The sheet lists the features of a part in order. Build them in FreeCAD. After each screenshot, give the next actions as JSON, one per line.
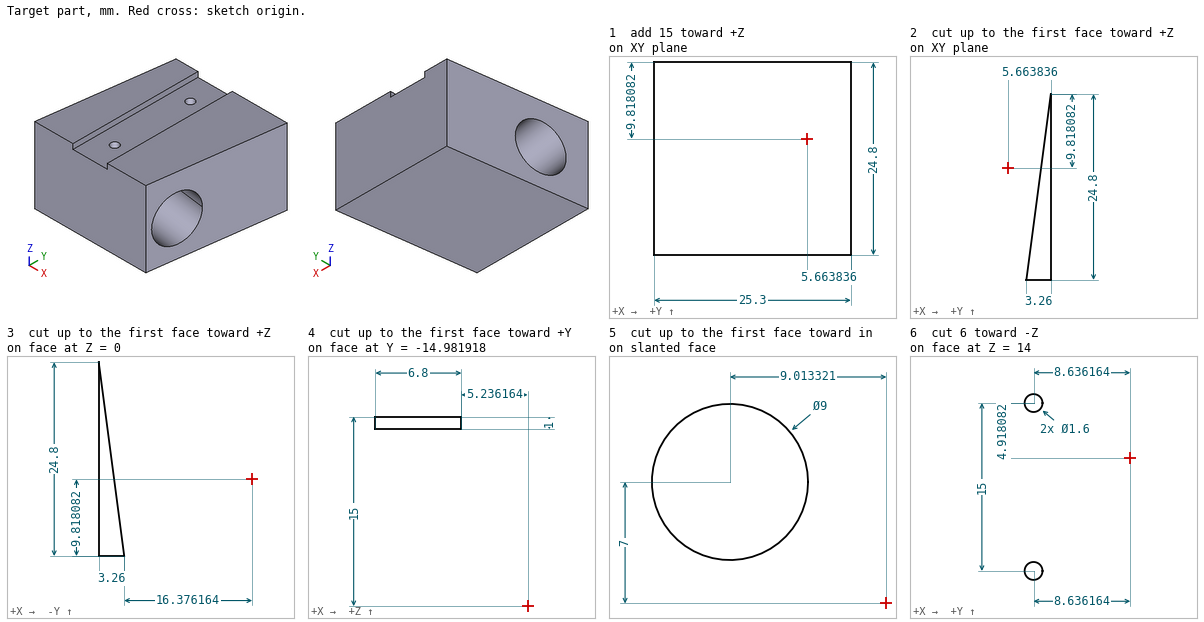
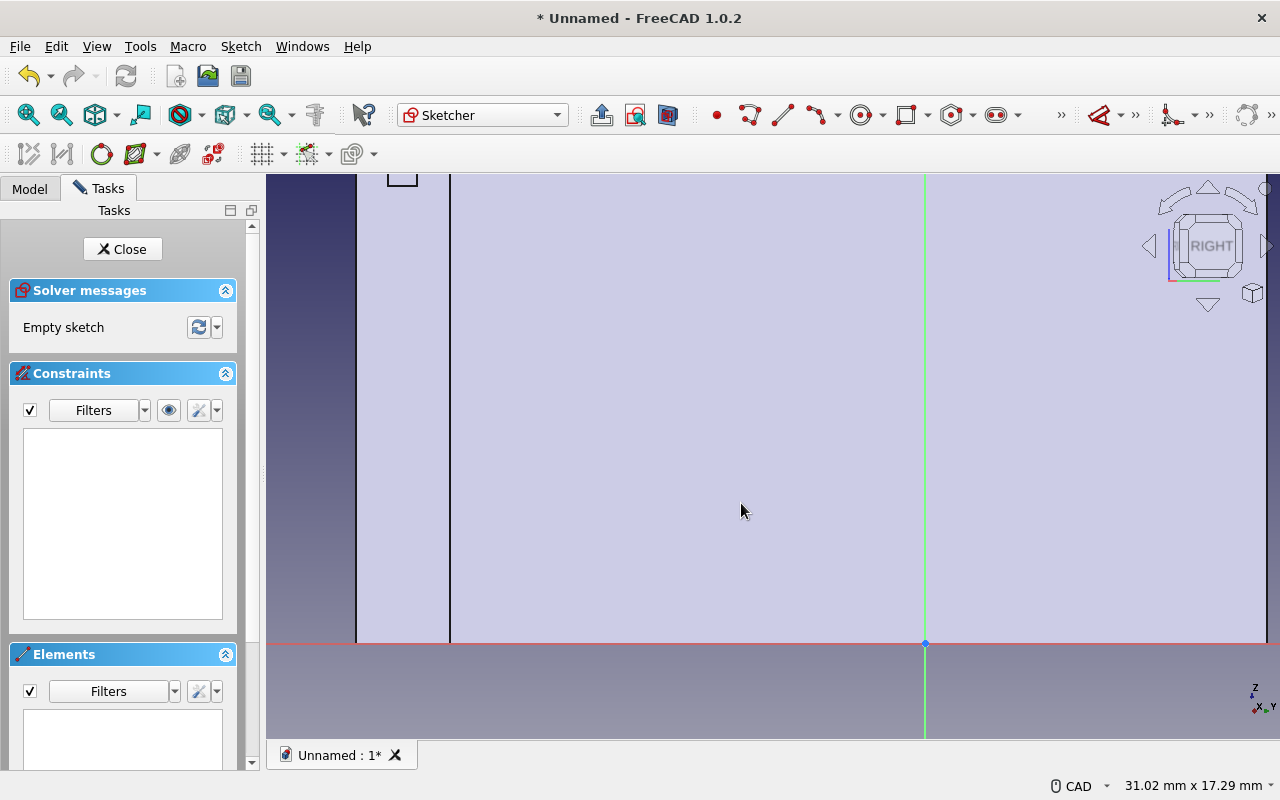
{"action": "left_click", "coordinate": [860, 116]}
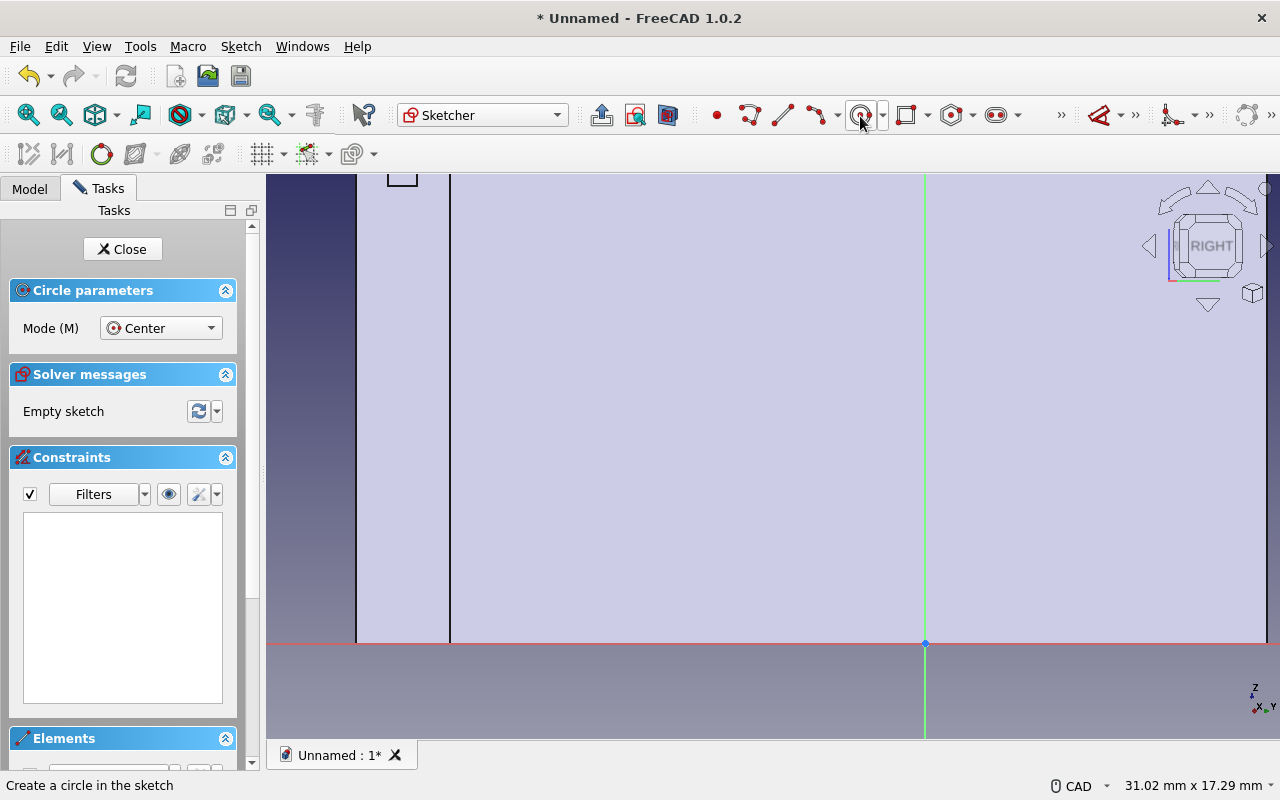
{"action": "left_click", "coordinate": [630, 415]}
{"action": "mouse_move", "coordinate": [734, 311]}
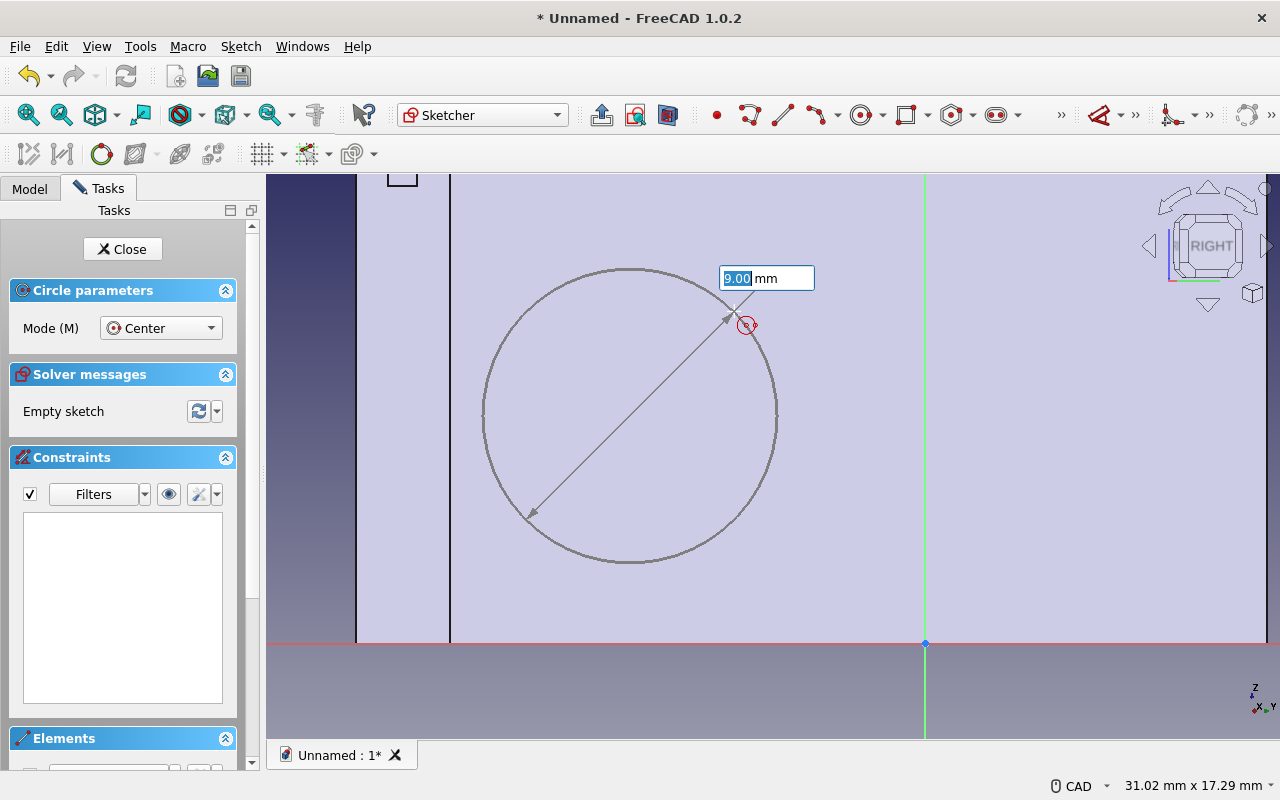
{"action": "type", "text": "9"}
{"action": "key", "text": "Return"}
{"action": "key", "text": "Escape"}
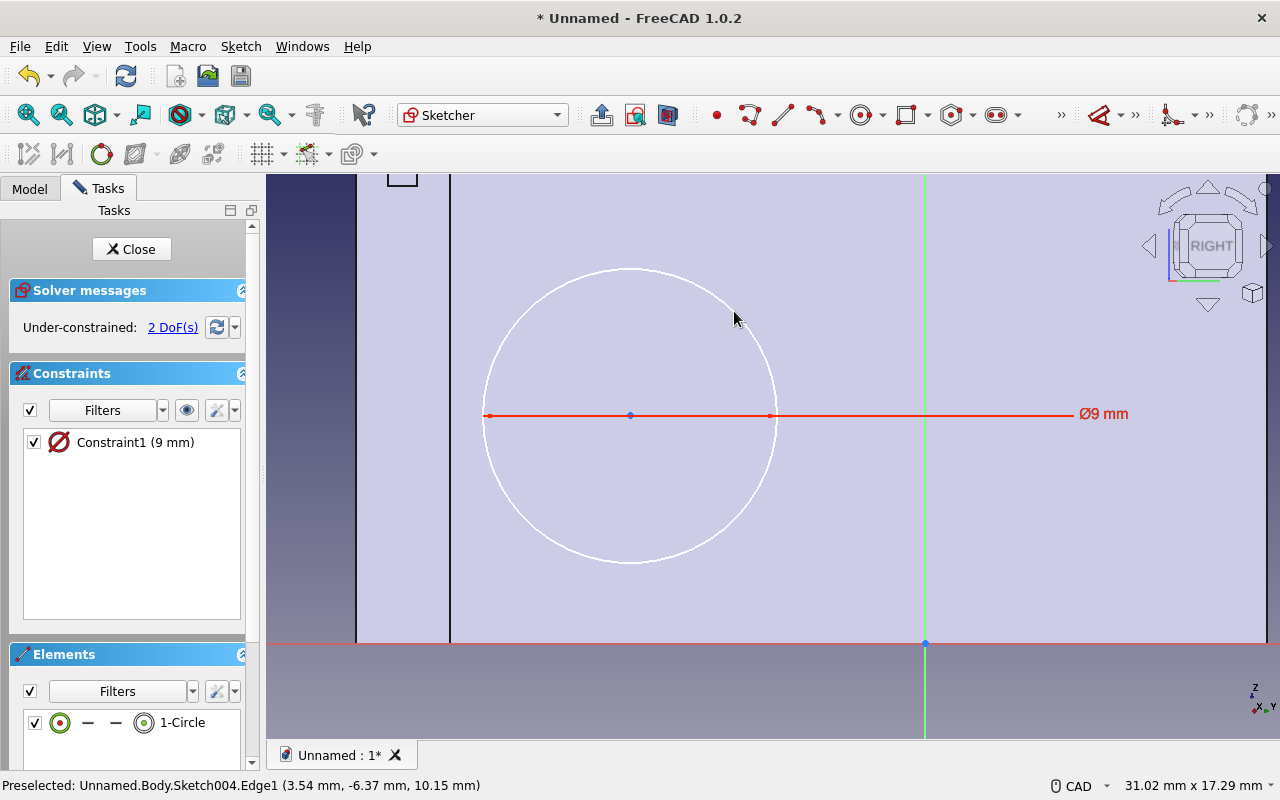
{"action": "left_click", "coordinate": [1098, 116]}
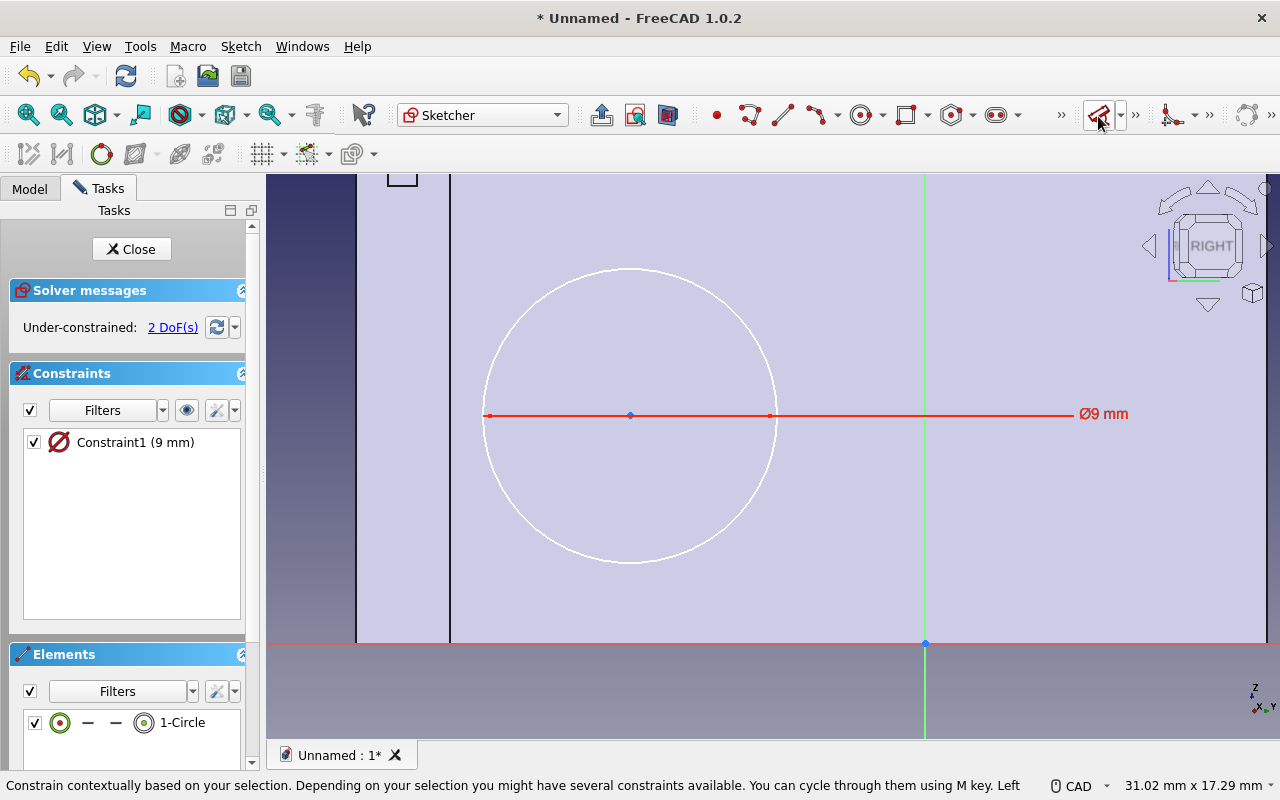
{"action": "left_click", "coordinate": [630, 416]}
{"action": "left_click", "coordinate": [959, 530]}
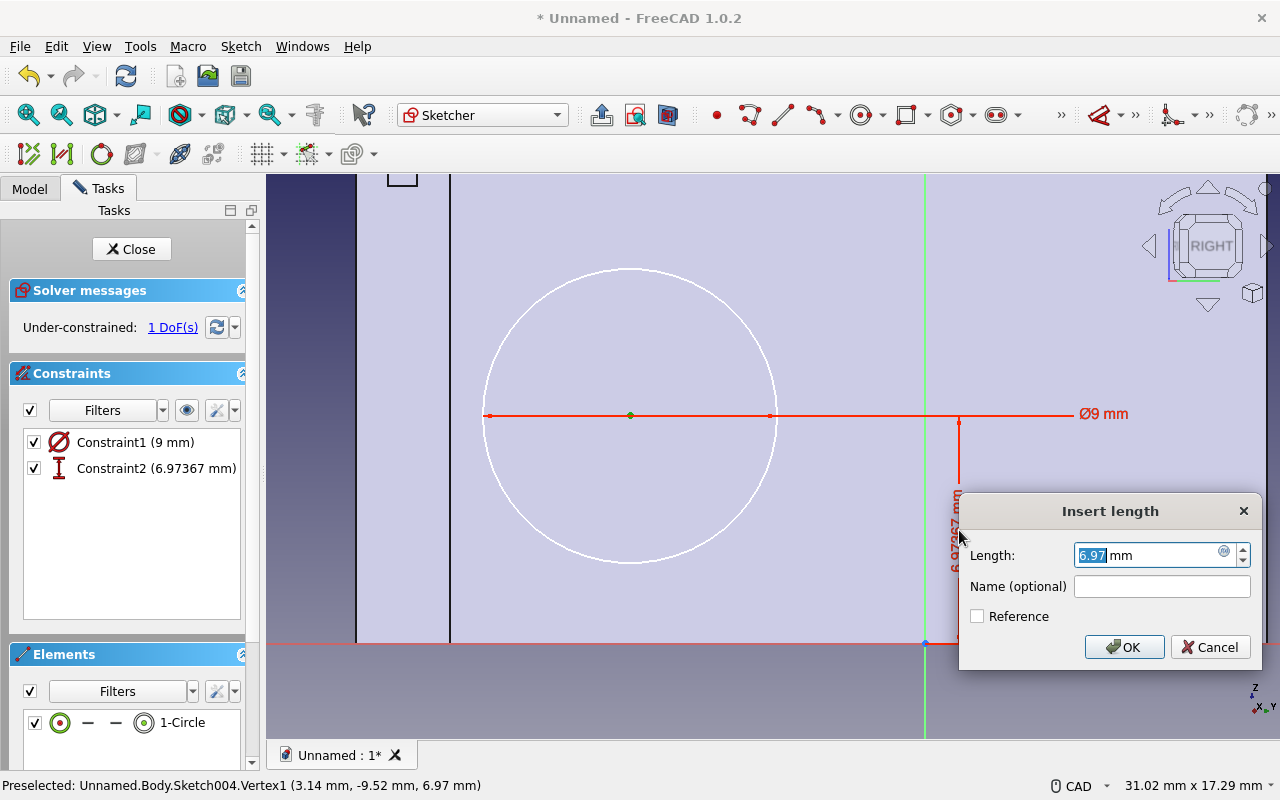
{"action": "type", "text": "7"}
{"action": "key", "text": "Return"}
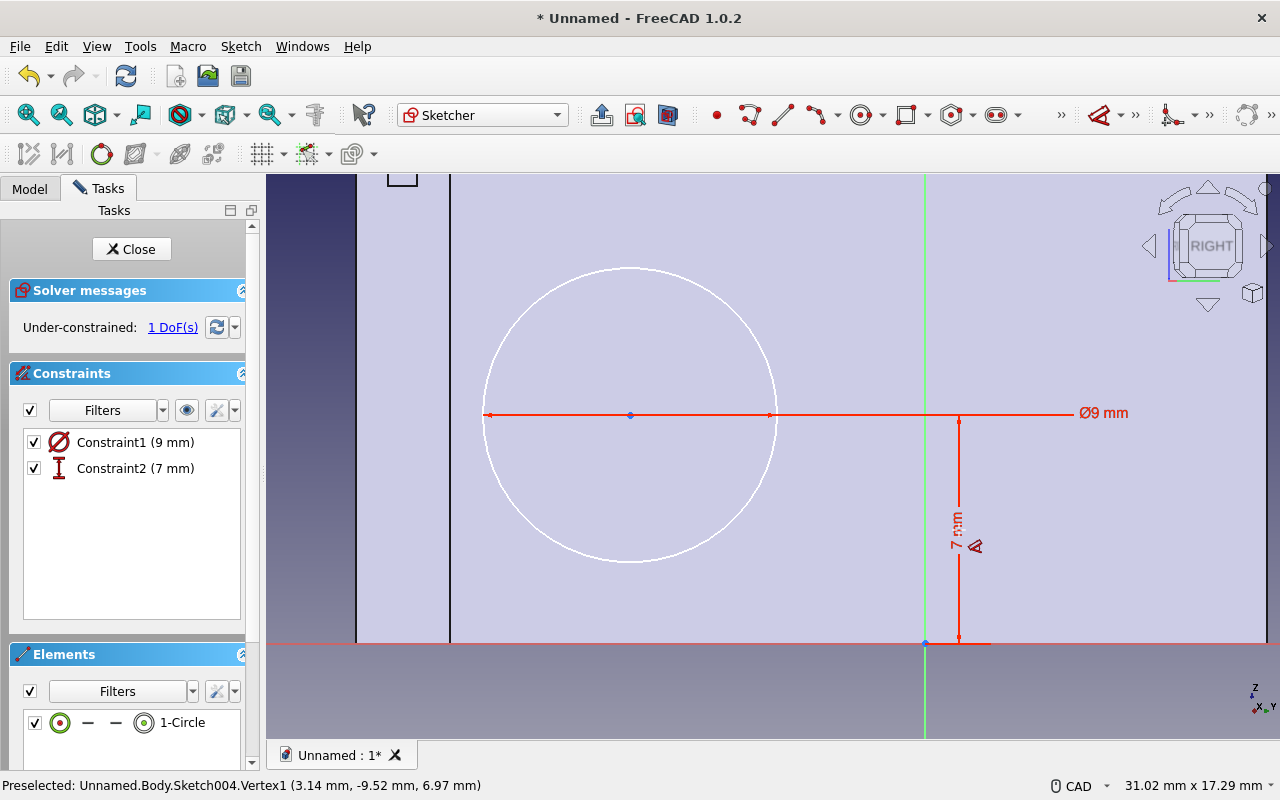
{"action": "left_click", "coordinate": [630, 415]}
{"action": "left_click", "coordinate": [778, 678]}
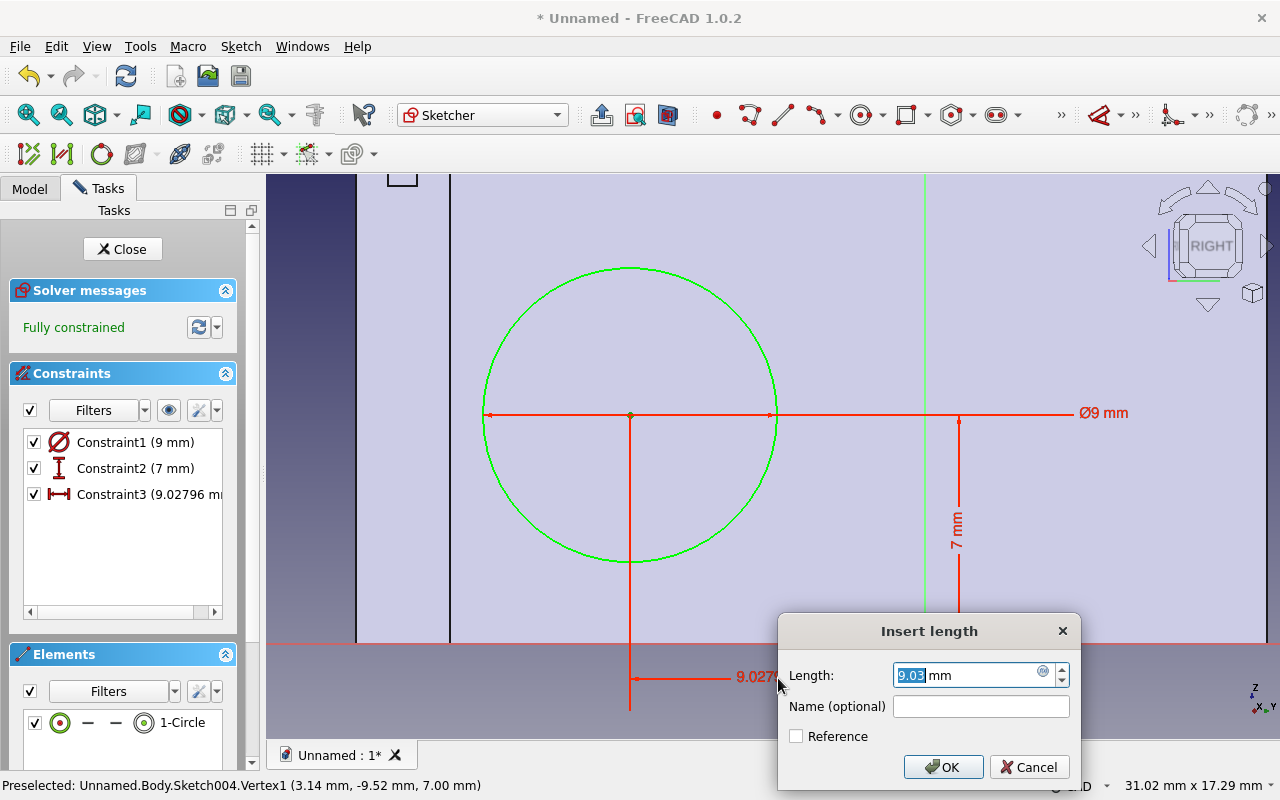
{"action": "type", "text": "9.013321"}
{"action": "key", "text": "Return"}
{"action": "key", "text": "Escape"}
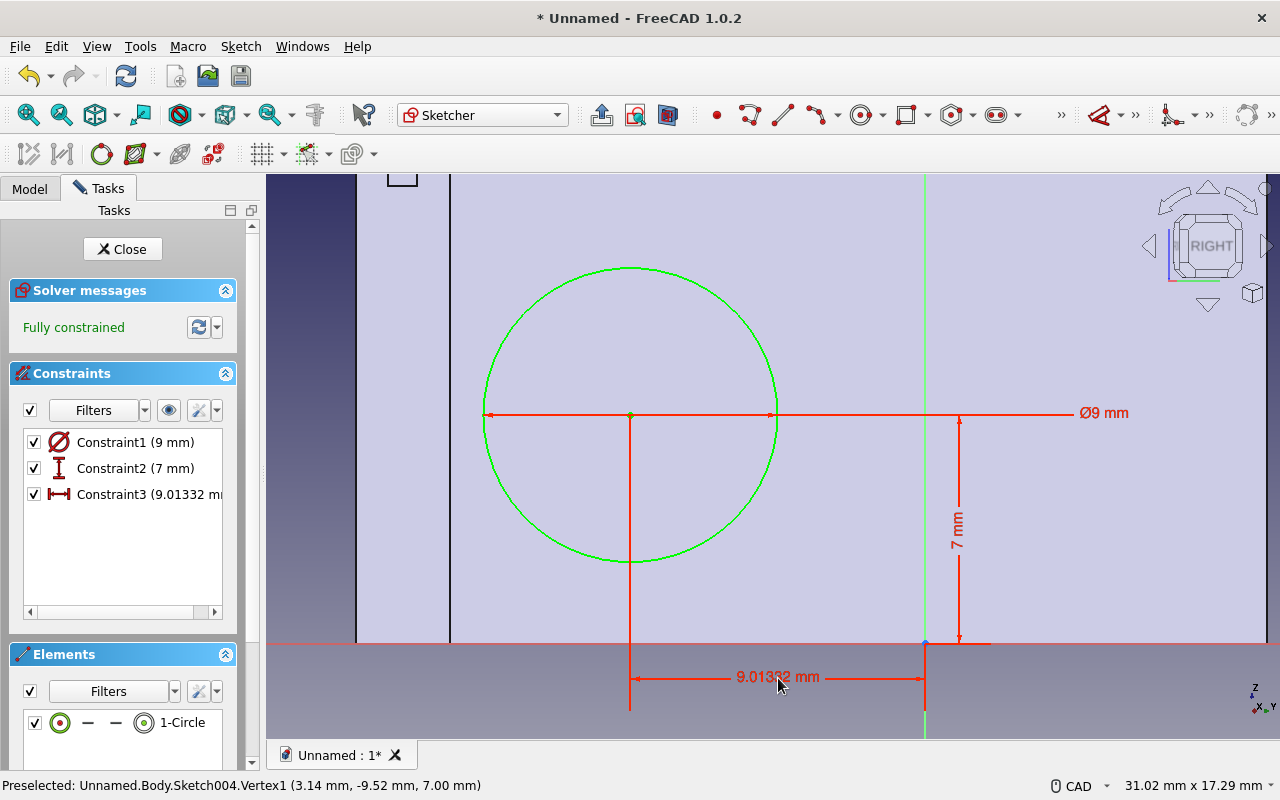
{"action": "left_click", "coordinate": [123, 249]}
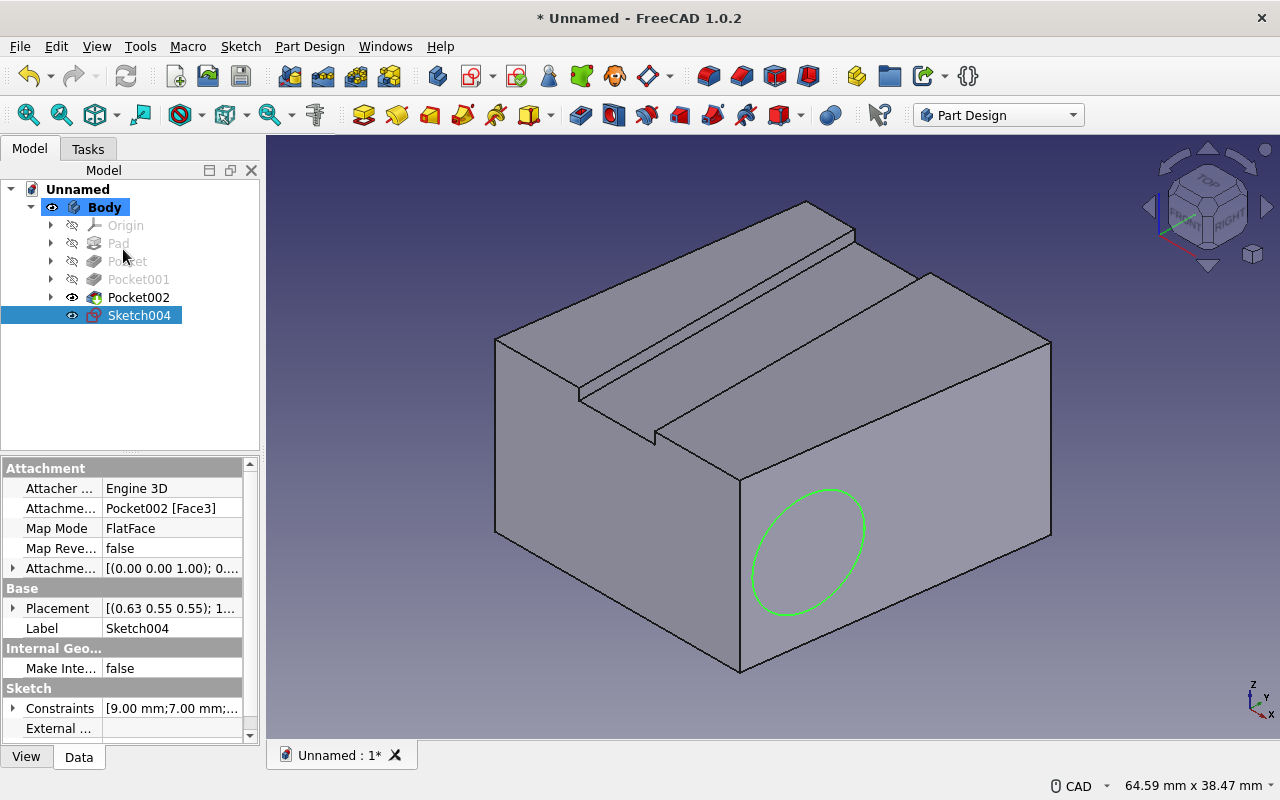
{"action": "left_click", "coordinate": [581, 116]}